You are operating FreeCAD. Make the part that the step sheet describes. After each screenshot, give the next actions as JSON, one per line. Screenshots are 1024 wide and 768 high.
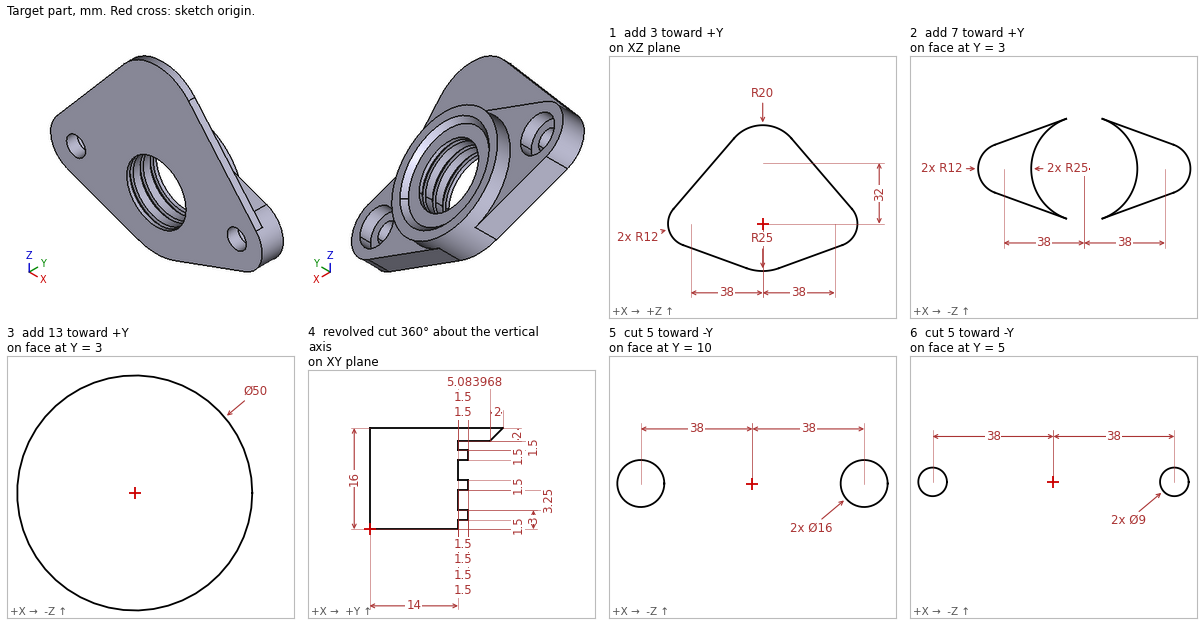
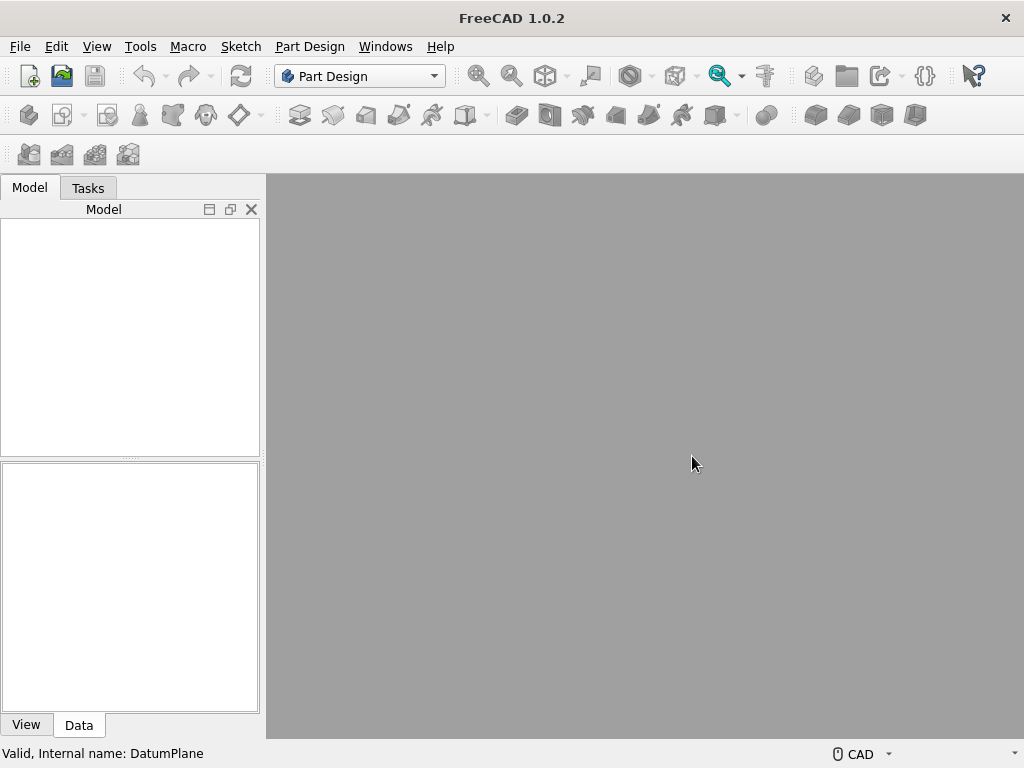
{"action": "left_click", "coordinate": [29, 76]}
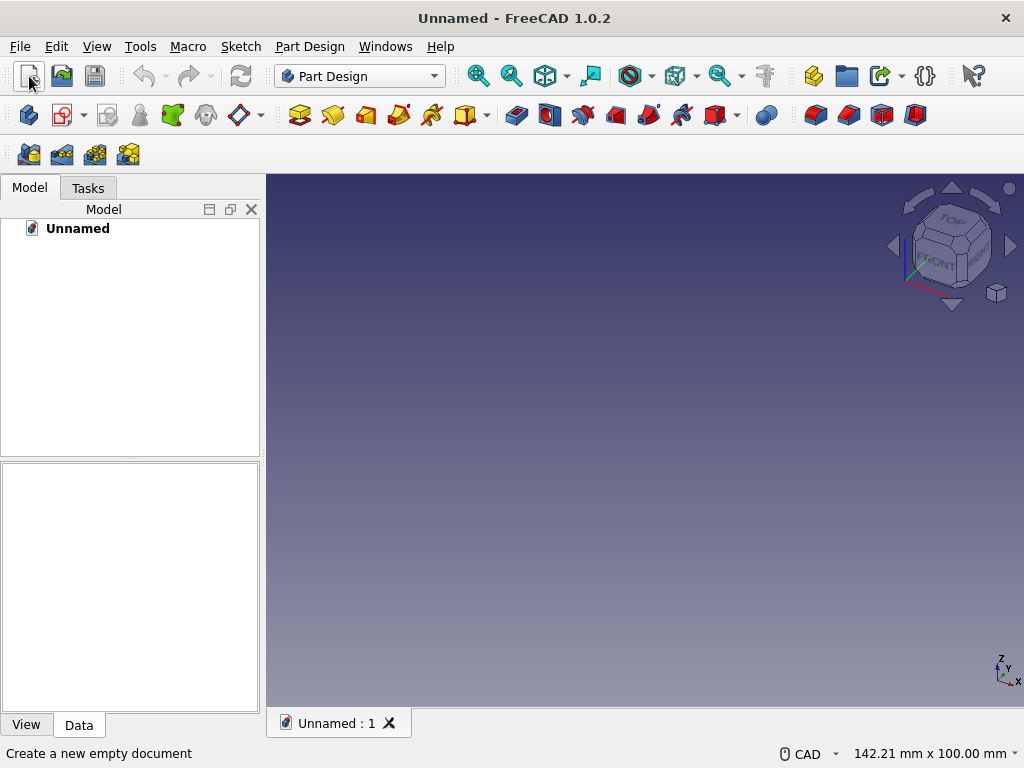
{"action": "left_click", "coordinate": [62, 116]}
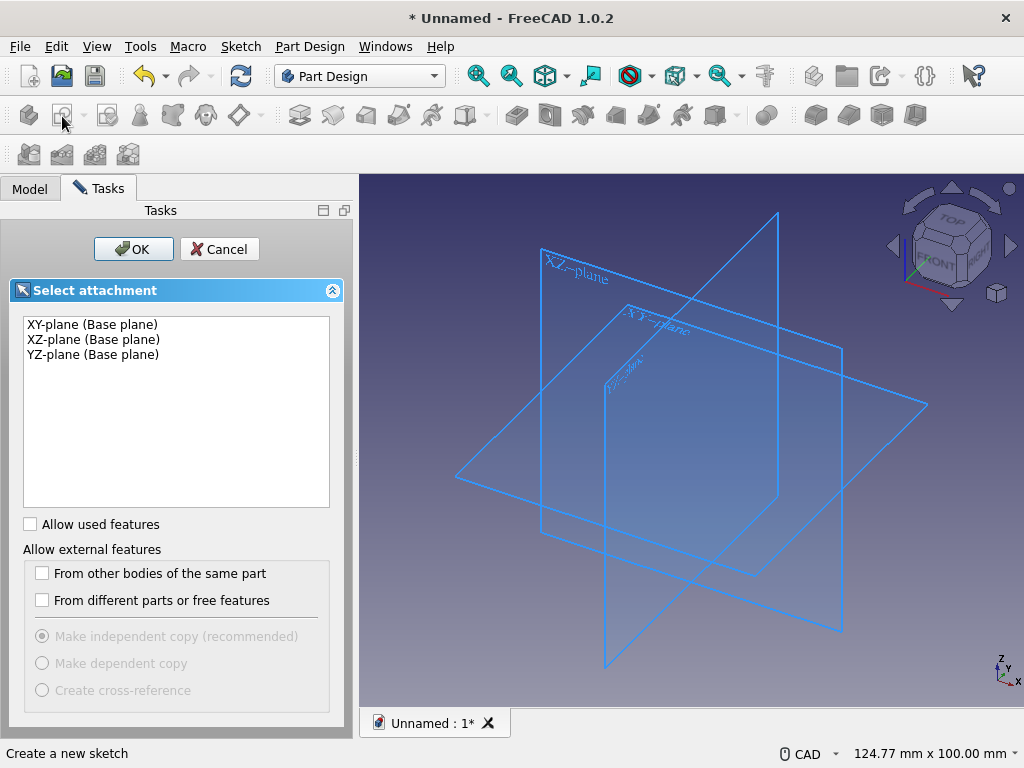
{"action": "left_click", "coordinate": [84, 340]}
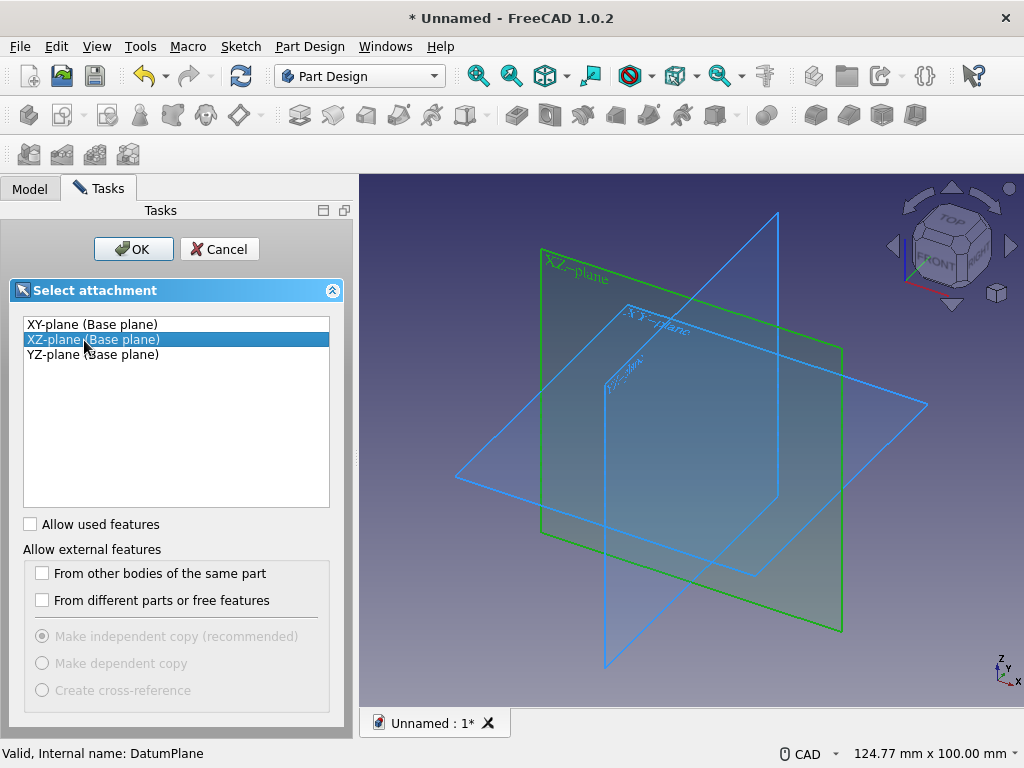
{"action": "left_click", "coordinate": [134, 249]}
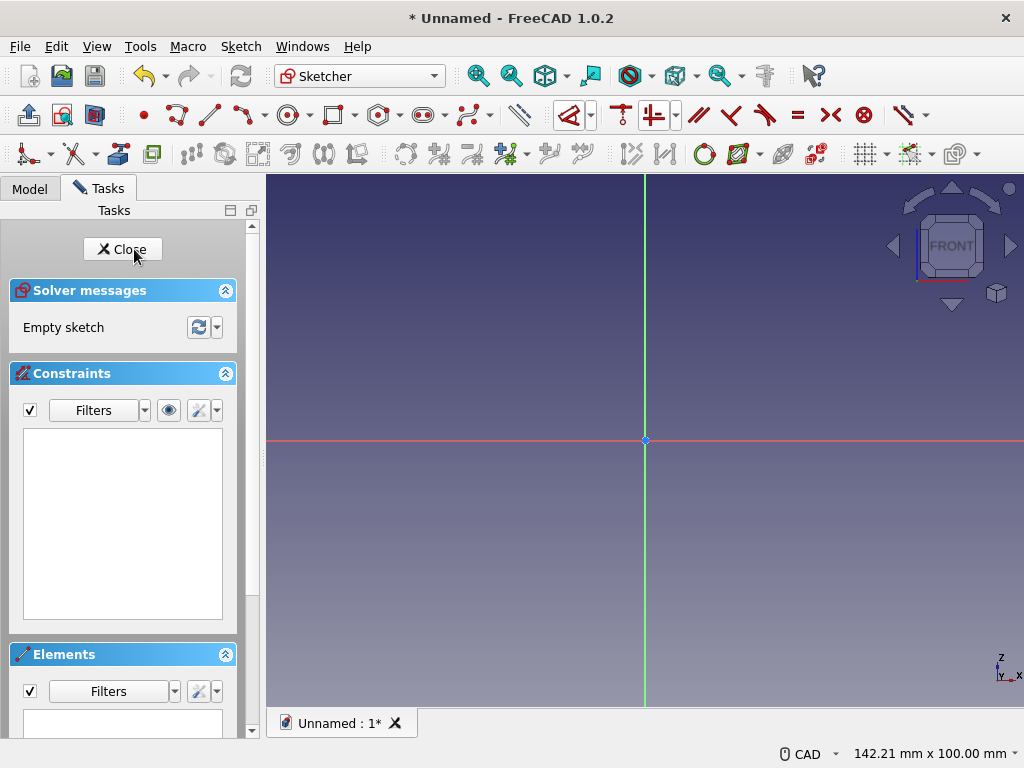
{"action": "scroll", "coordinate": [294, 679], "scroll_direction": "down", "scroll_amount": 1}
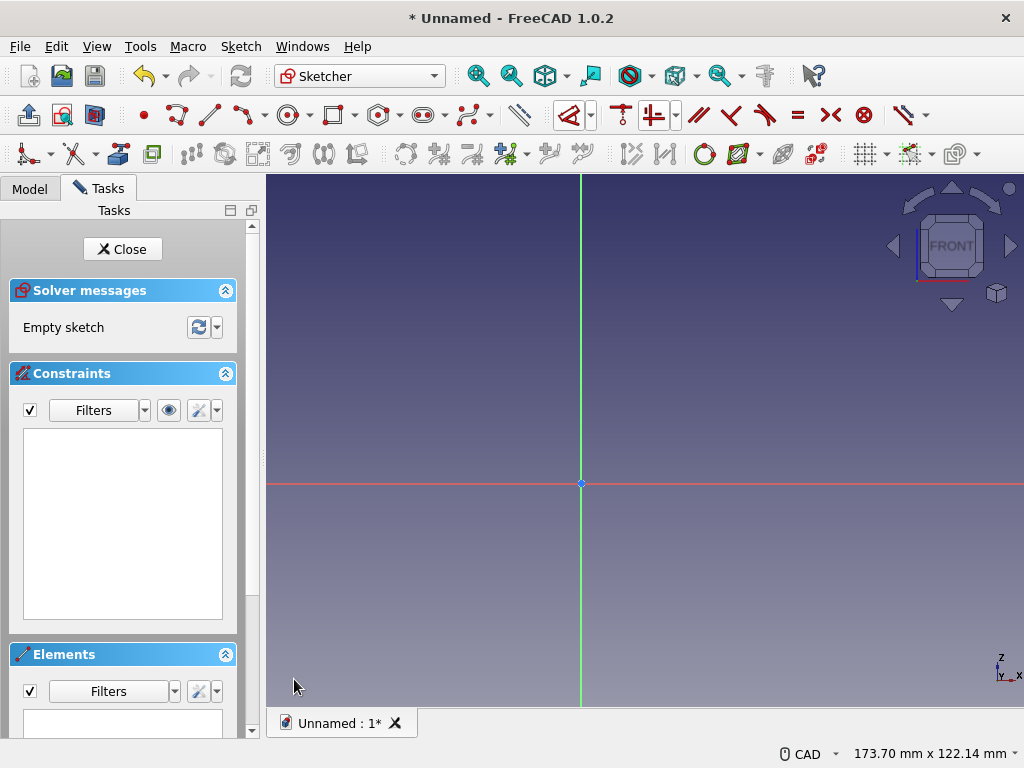
{"action": "left_click", "coordinate": [210, 116]}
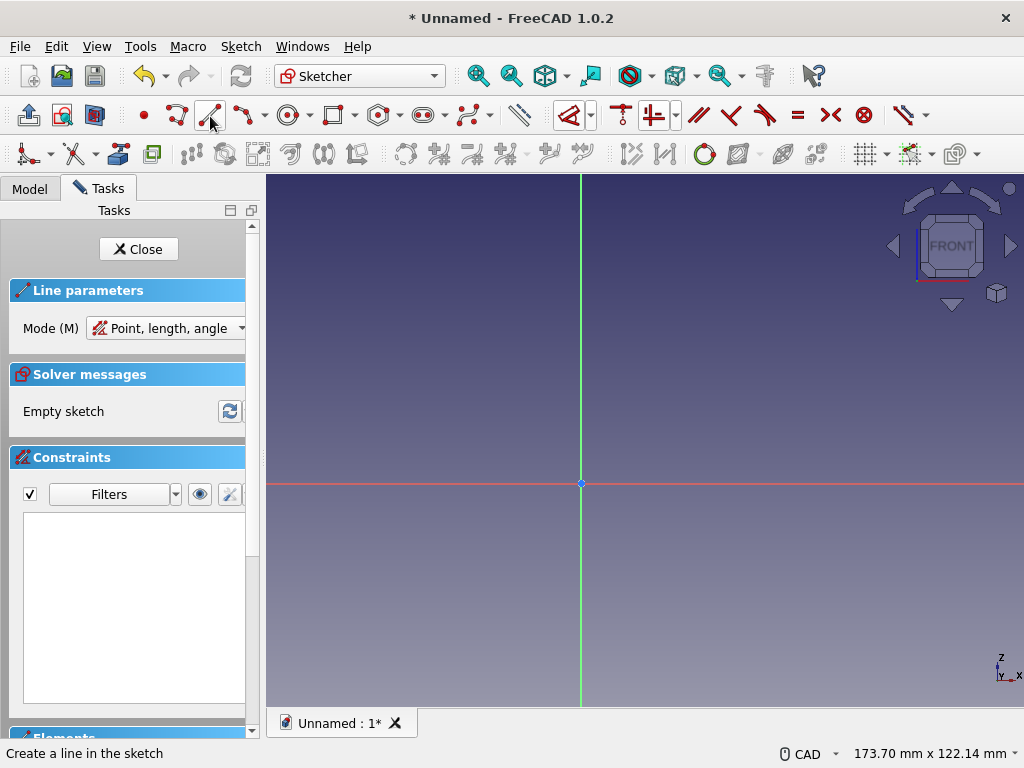
{"action": "left_click", "coordinate": [544, 586]}
{"action": "left_click", "coordinate": [398, 533]}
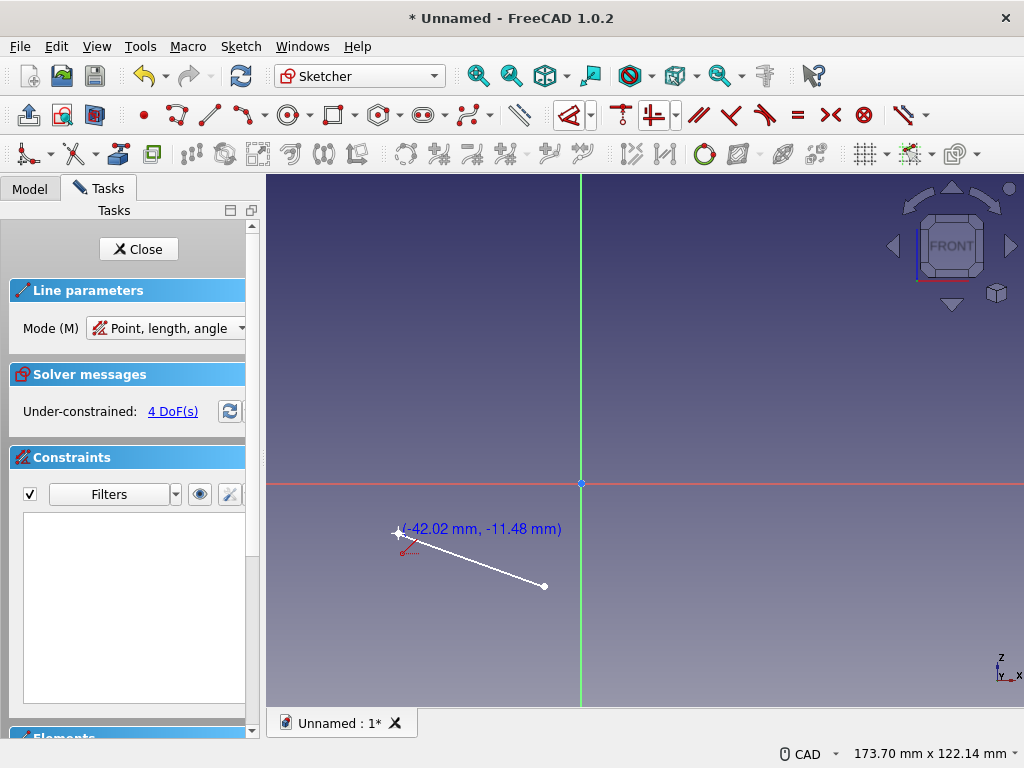
{"action": "left_click", "coordinate": [376, 450]}
{"action": "left_click", "coordinate": [515, 287]}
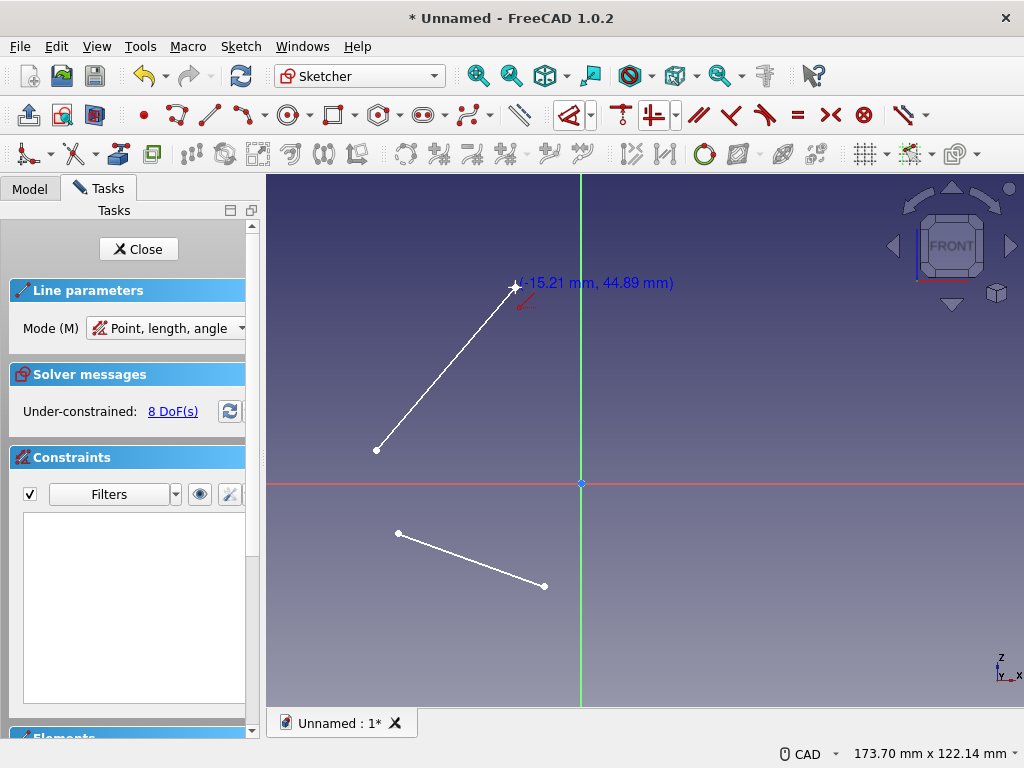
{"action": "left_click", "coordinate": [648, 287]}
{"action": "left_click", "coordinate": [787, 450]}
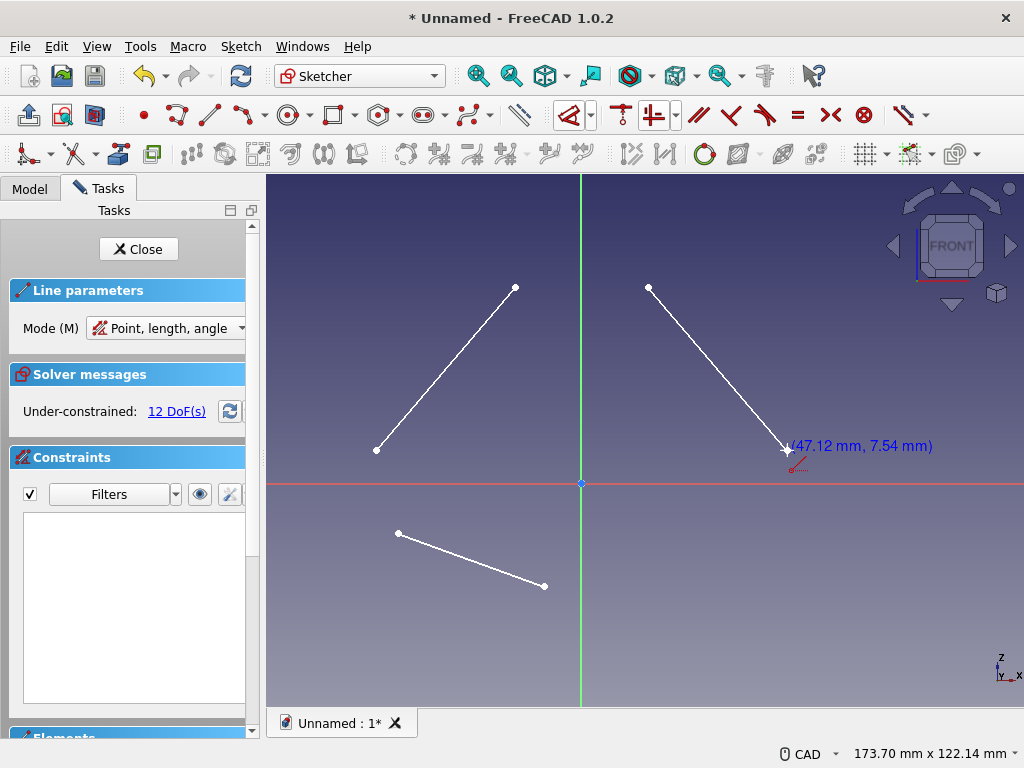
{"action": "left_click", "coordinate": [765, 533]}
{"action": "left_click", "coordinate": [619, 586]}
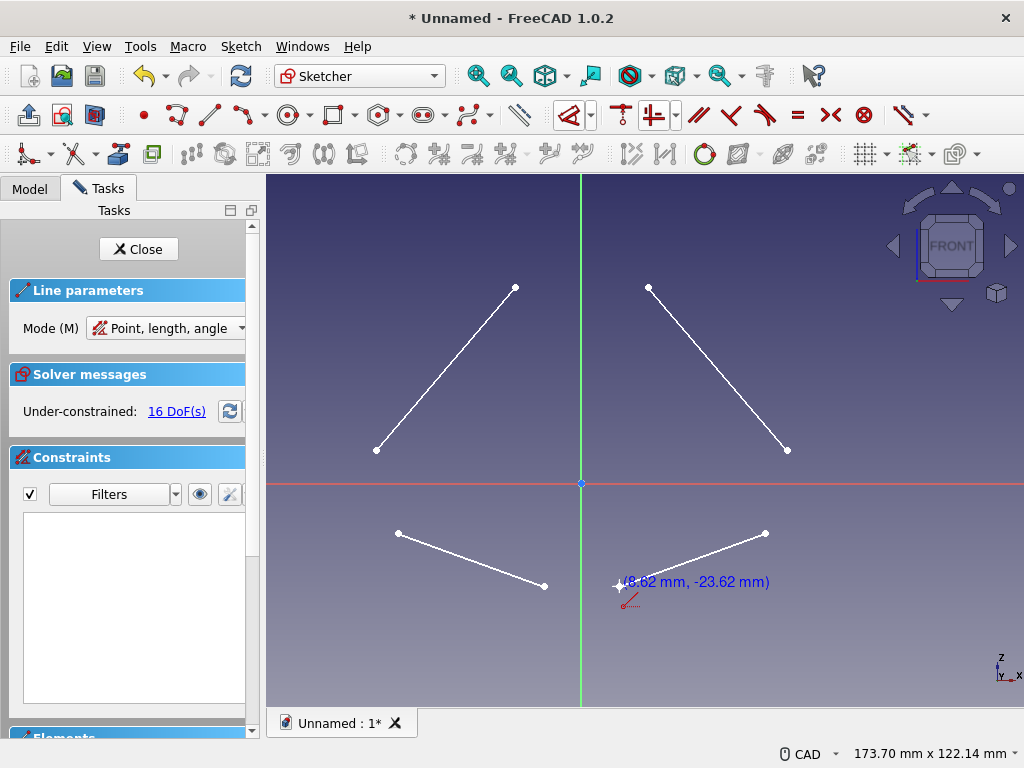
{"action": "left_click", "coordinate": [242, 116]}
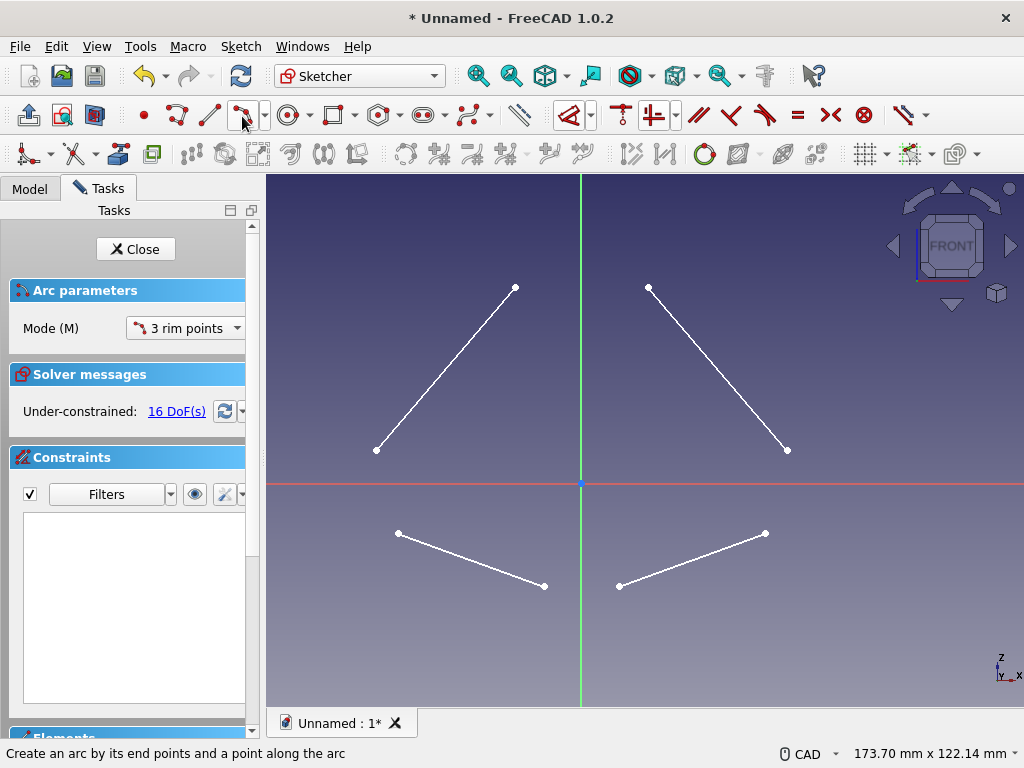
{"action": "left_click", "coordinate": [398, 534]}
{"action": "left_click", "coordinate": [376, 451]}
{"action": "left_click", "coordinate": [368, 507]}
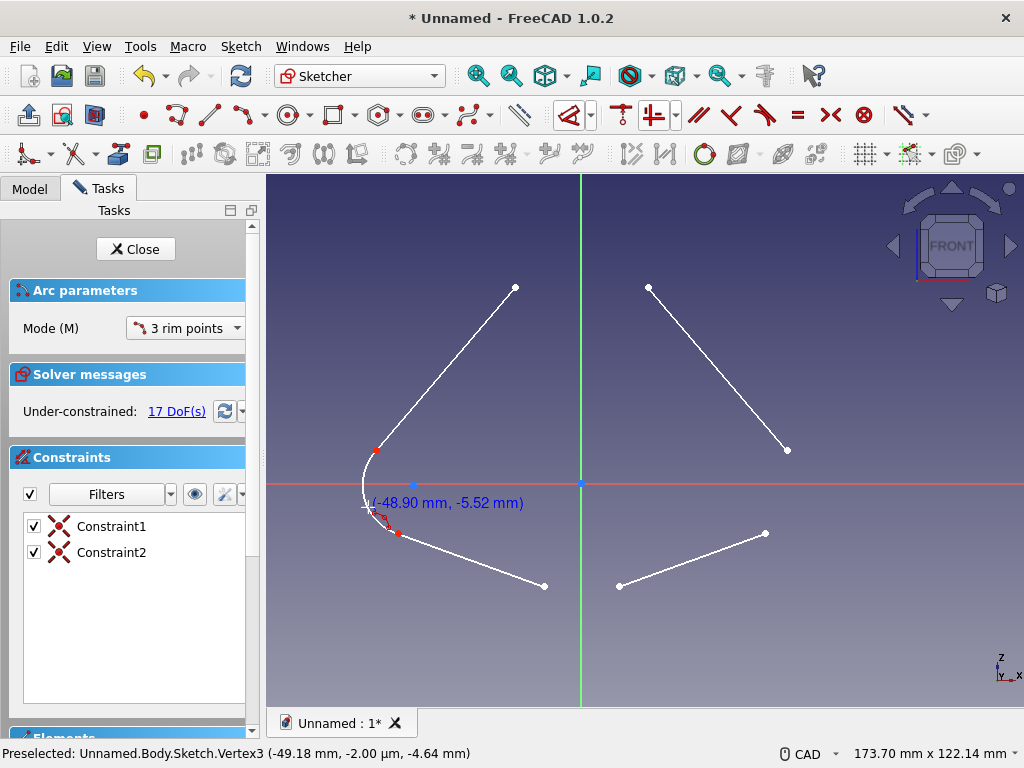
{"action": "left_click", "coordinate": [515, 288]}
{"action": "left_click", "coordinate": [648, 288]}
{"action": "left_click", "coordinate": [596, 258]}